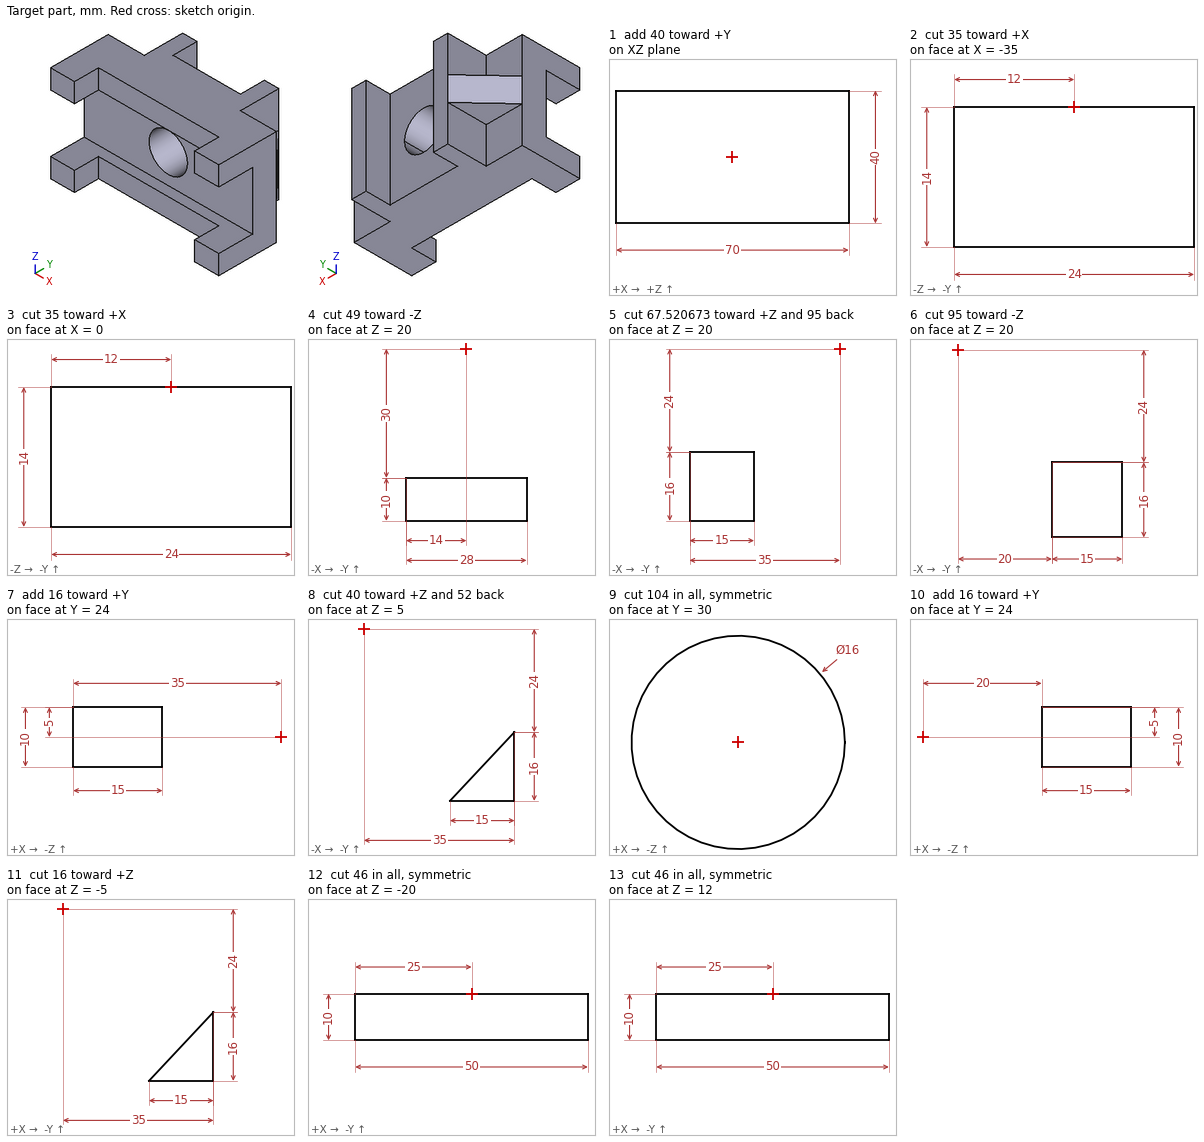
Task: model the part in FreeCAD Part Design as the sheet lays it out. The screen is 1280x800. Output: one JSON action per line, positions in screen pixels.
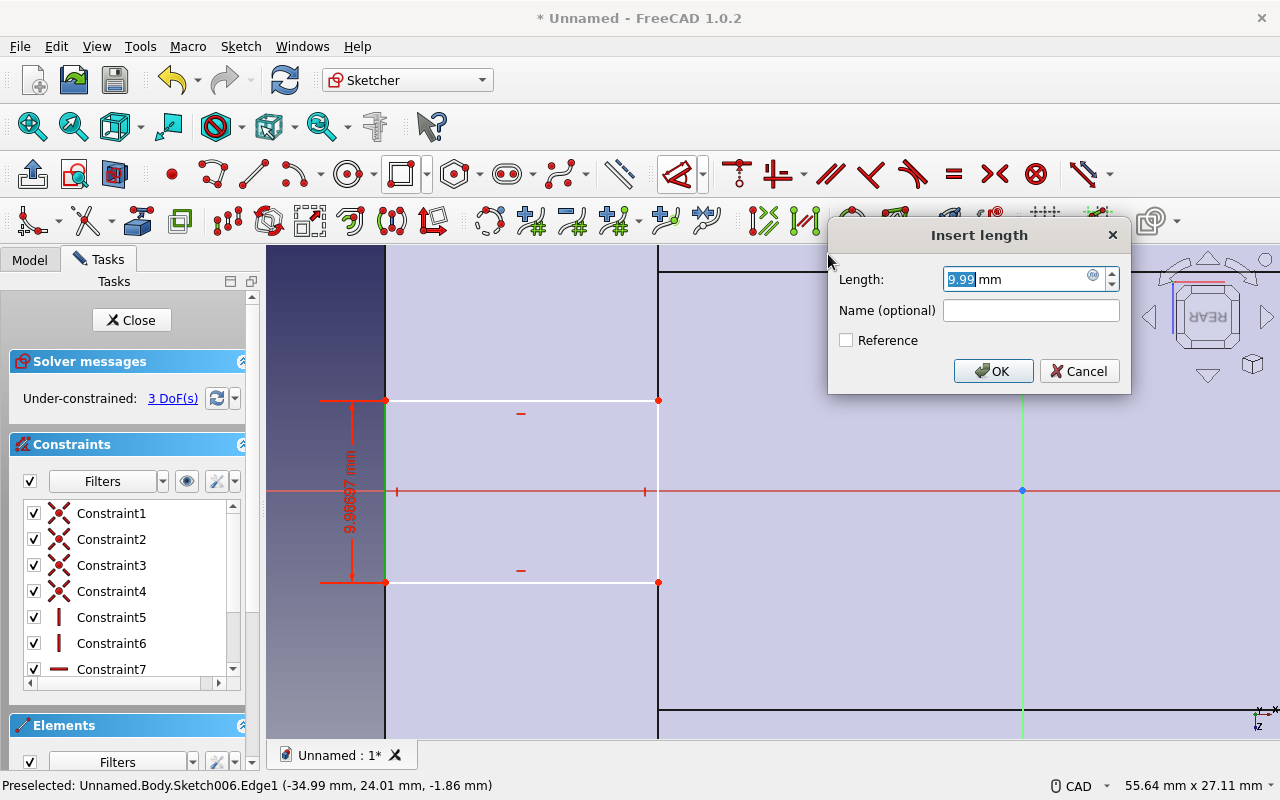
{"action": "type", "text": "10"}
{"action": "key", "text": "Return"}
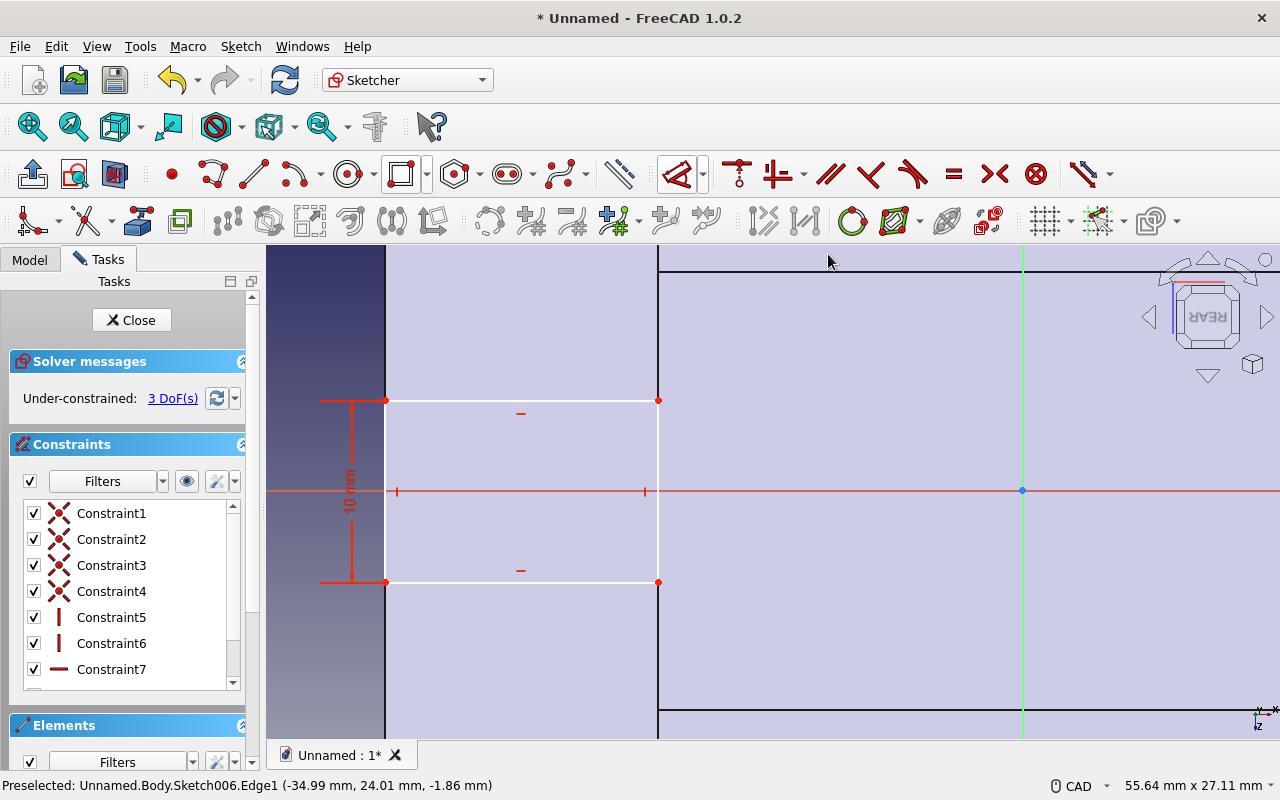
{"action": "left_click", "coordinate": [467, 583]}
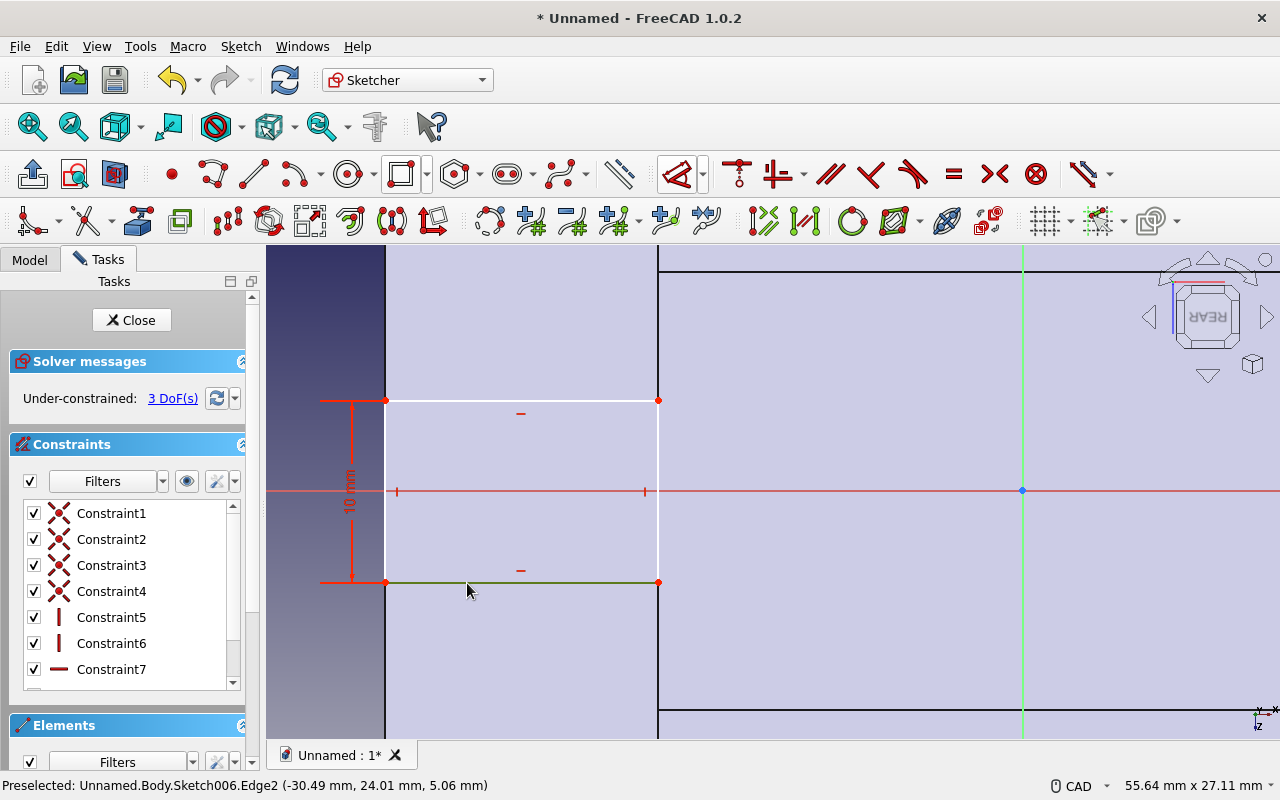
{"action": "key", "text": "l"}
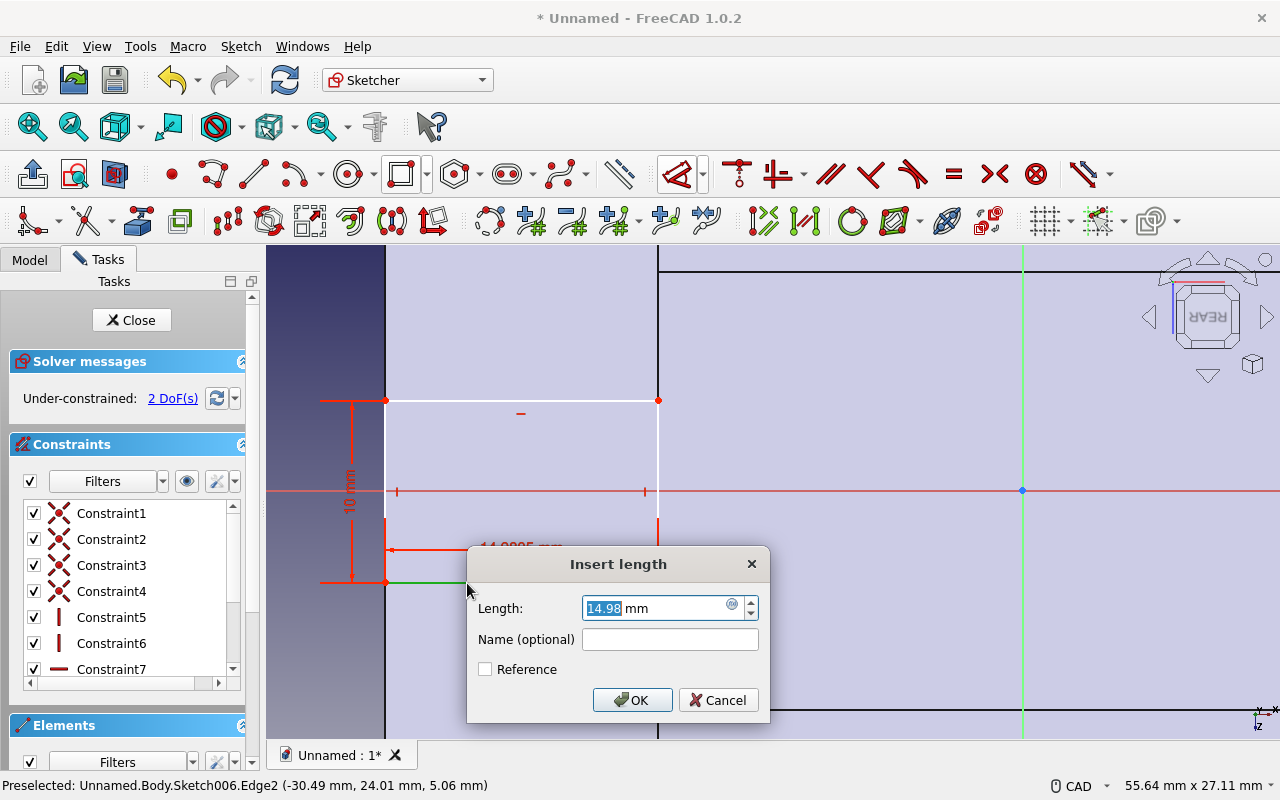
{"action": "type", "text": "15"}
{"action": "key", "text": "Return"}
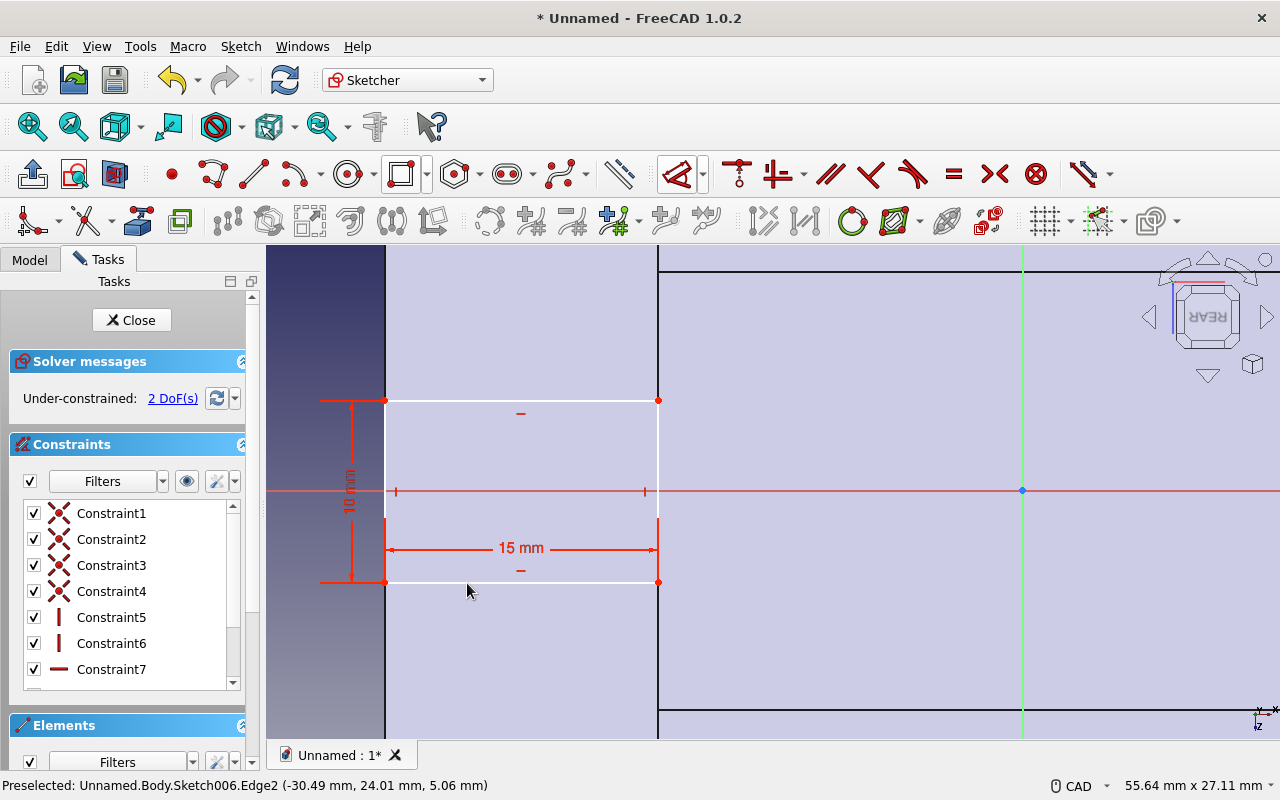
{"action": "left_click", "coordinate": [385, 401]}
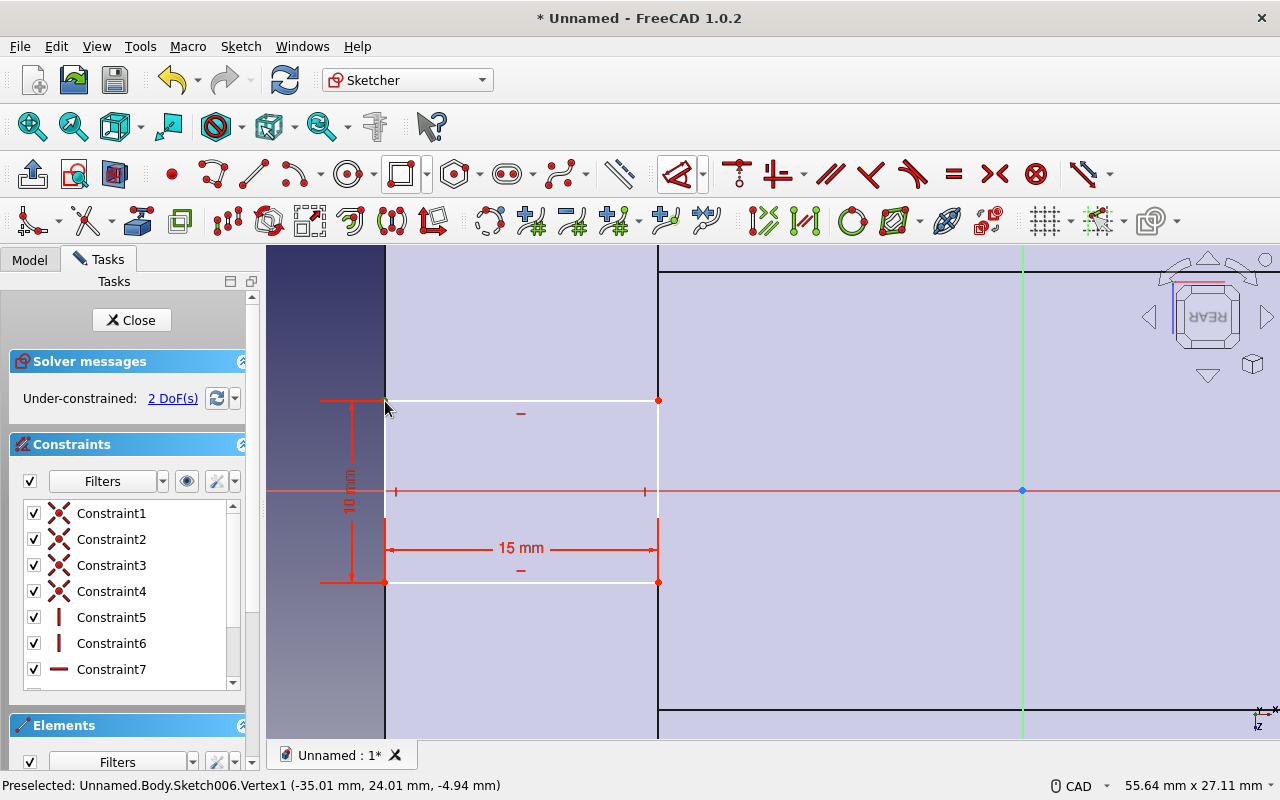
{"action": "key", "text": "i"}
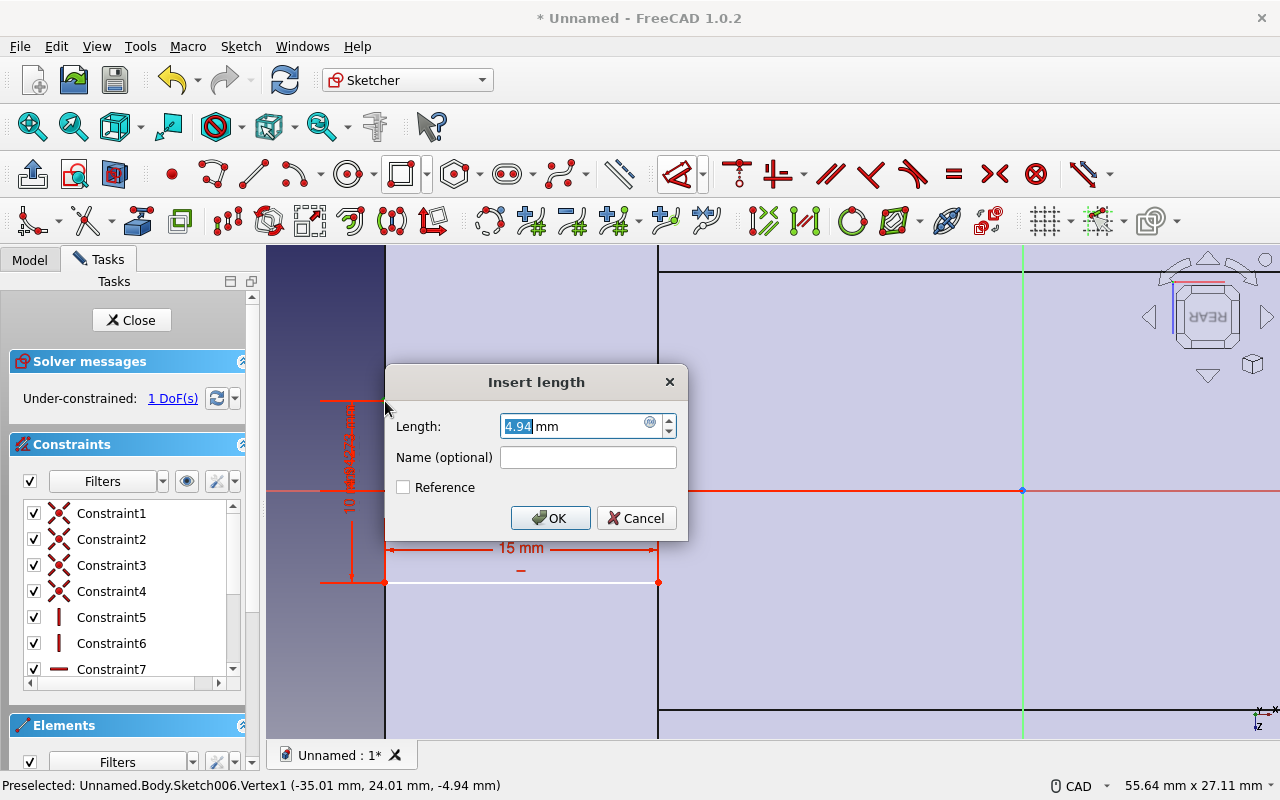
{"action": "type", "text": "5"}
{"action": "key", "text": "Return"}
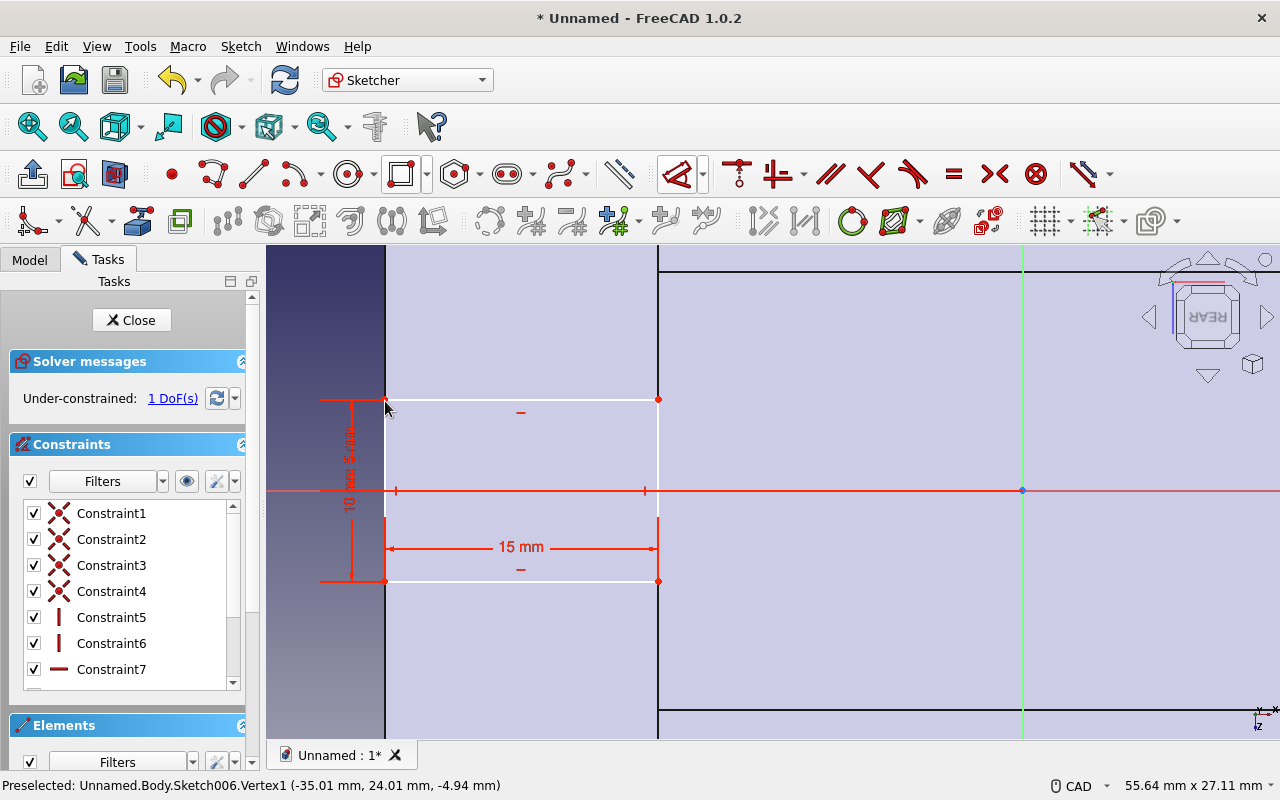
{"action": "left_click", "coordinate": [385, 400]}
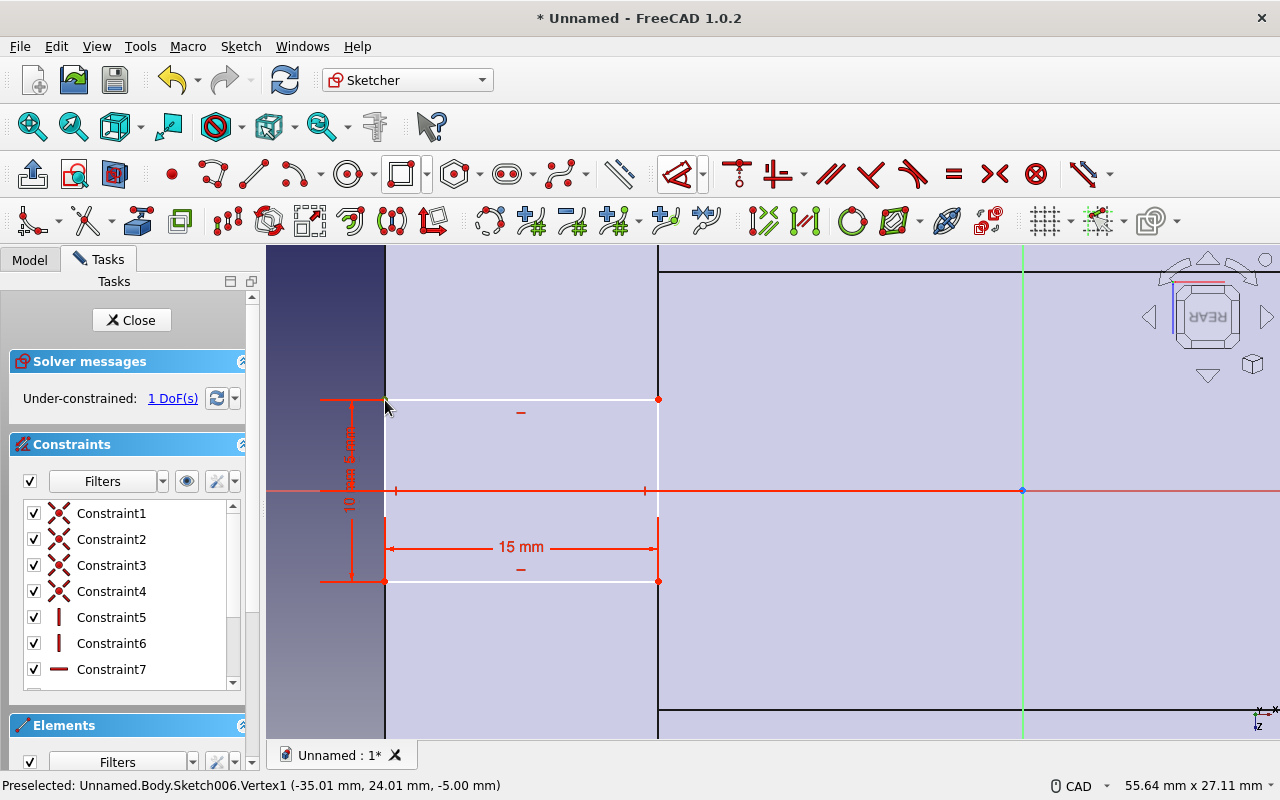
{"action": "key", "text": "l"}